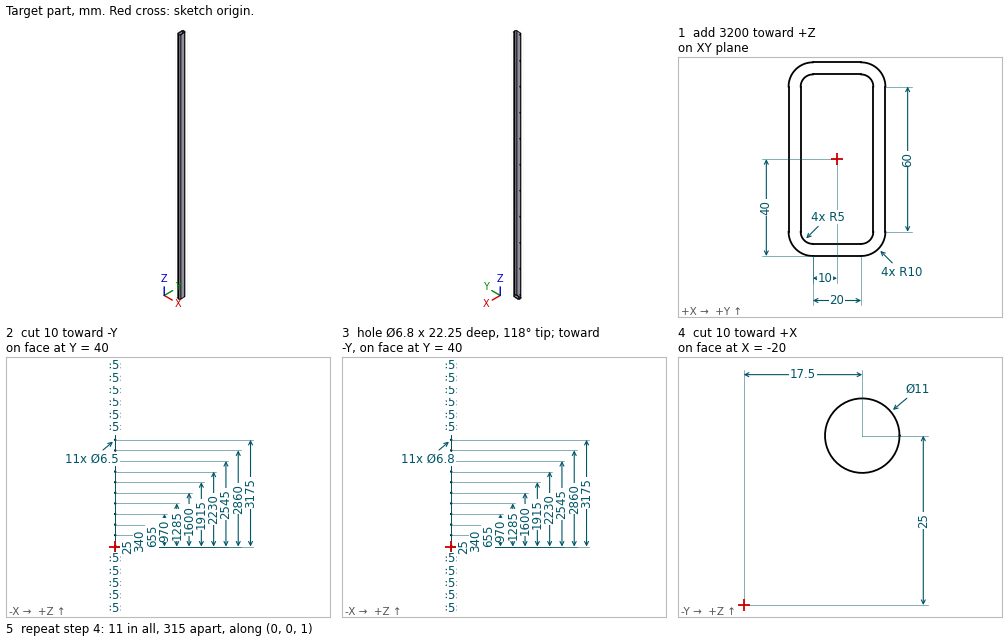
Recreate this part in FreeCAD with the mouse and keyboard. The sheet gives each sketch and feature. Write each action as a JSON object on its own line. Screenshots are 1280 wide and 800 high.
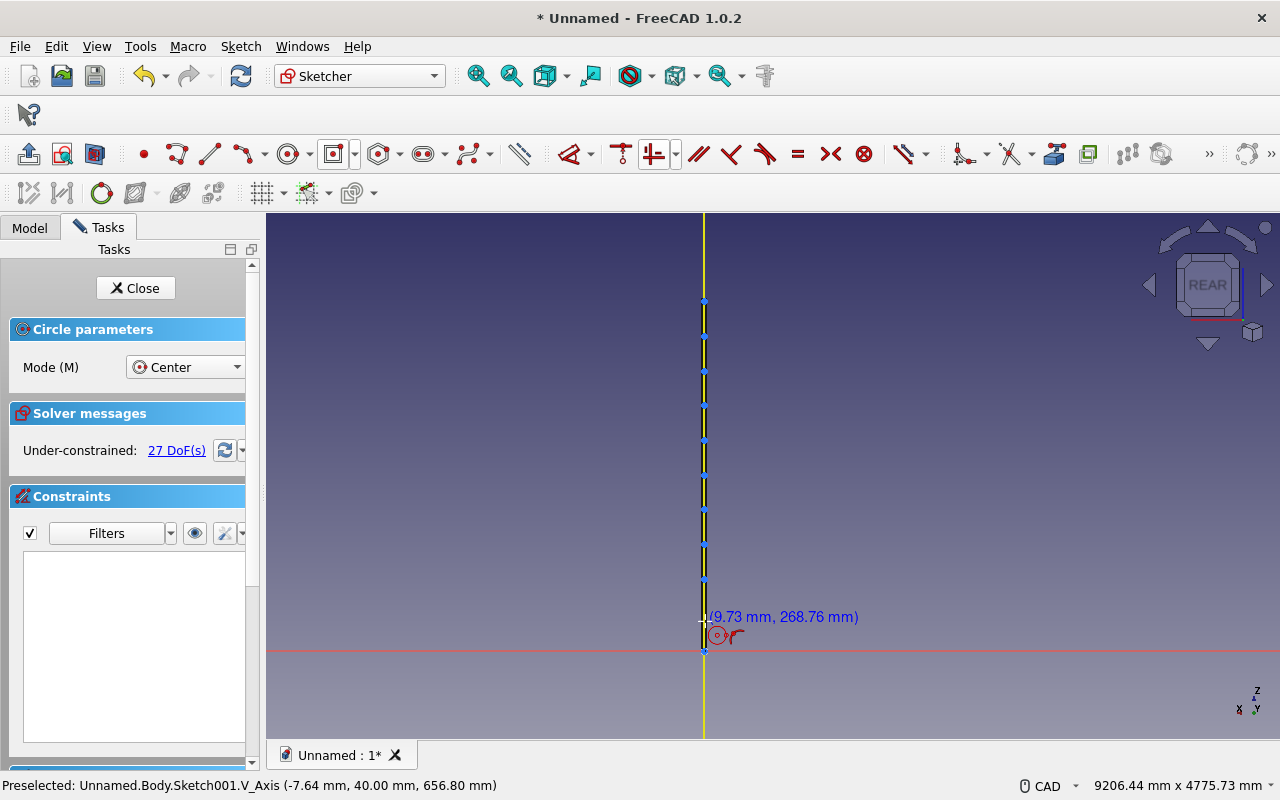
{"action": "scroll", "coordinate": [705, 614], "scroll_direction": "up", "scroll_amount": 21}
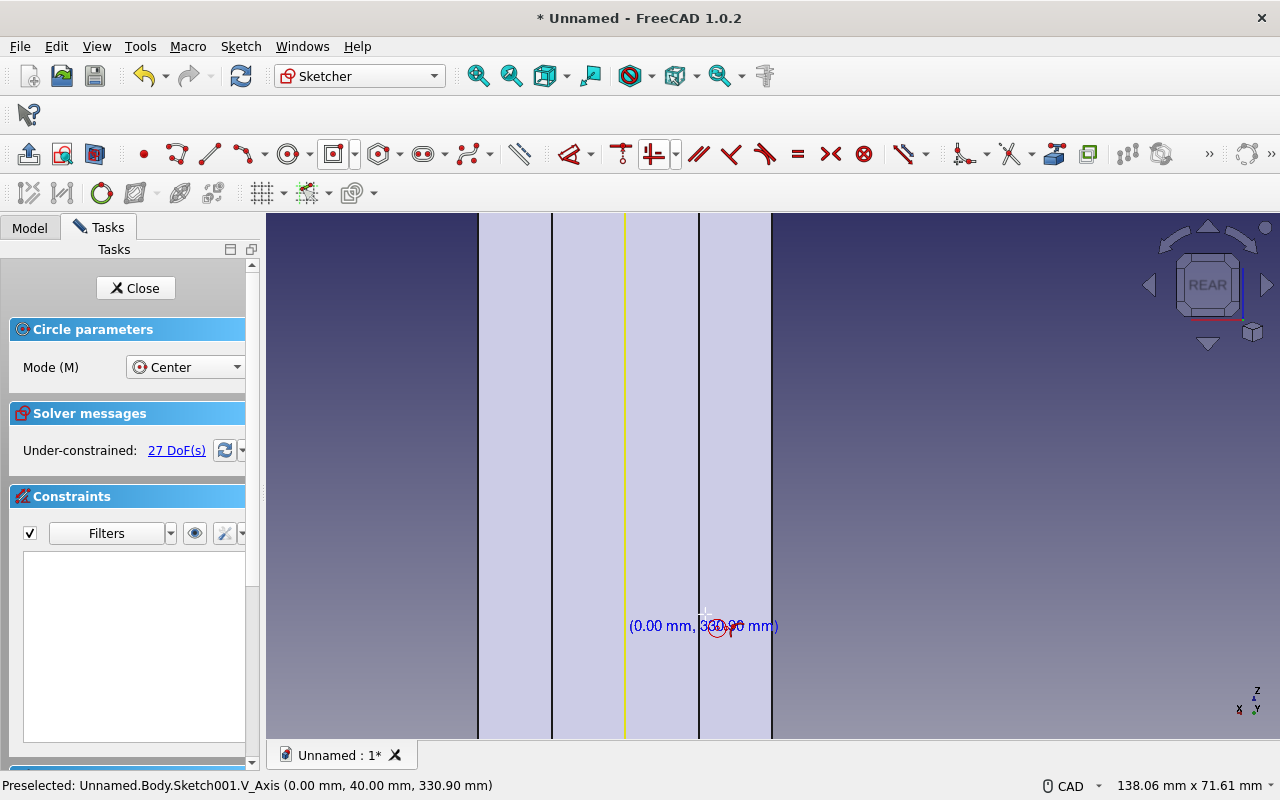
{"action": "left_click", "coordinate": [662, 564]}
{"action": "left_click", "coordinate": [679, 547]}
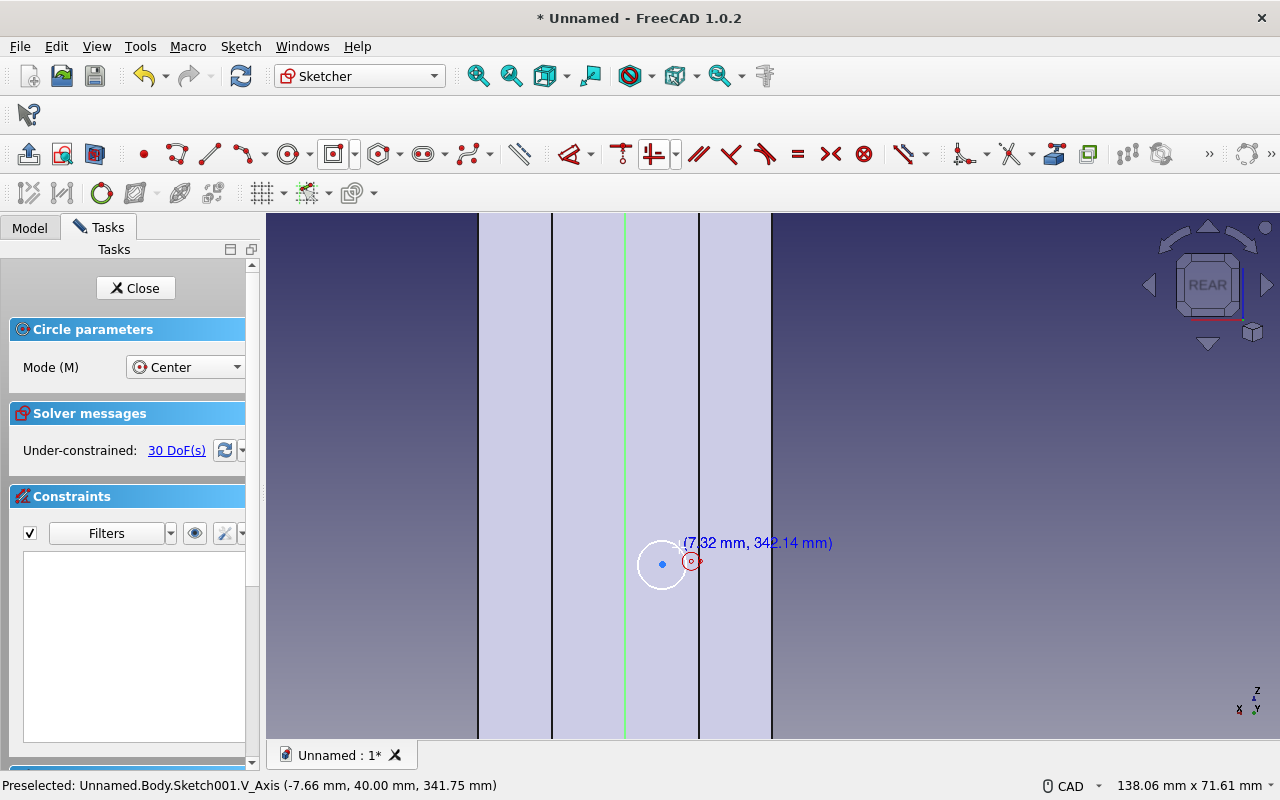
{"action": "scroll", "coordinate": [704, 476], "scroll_direction": "down", "scroll_amount": 15}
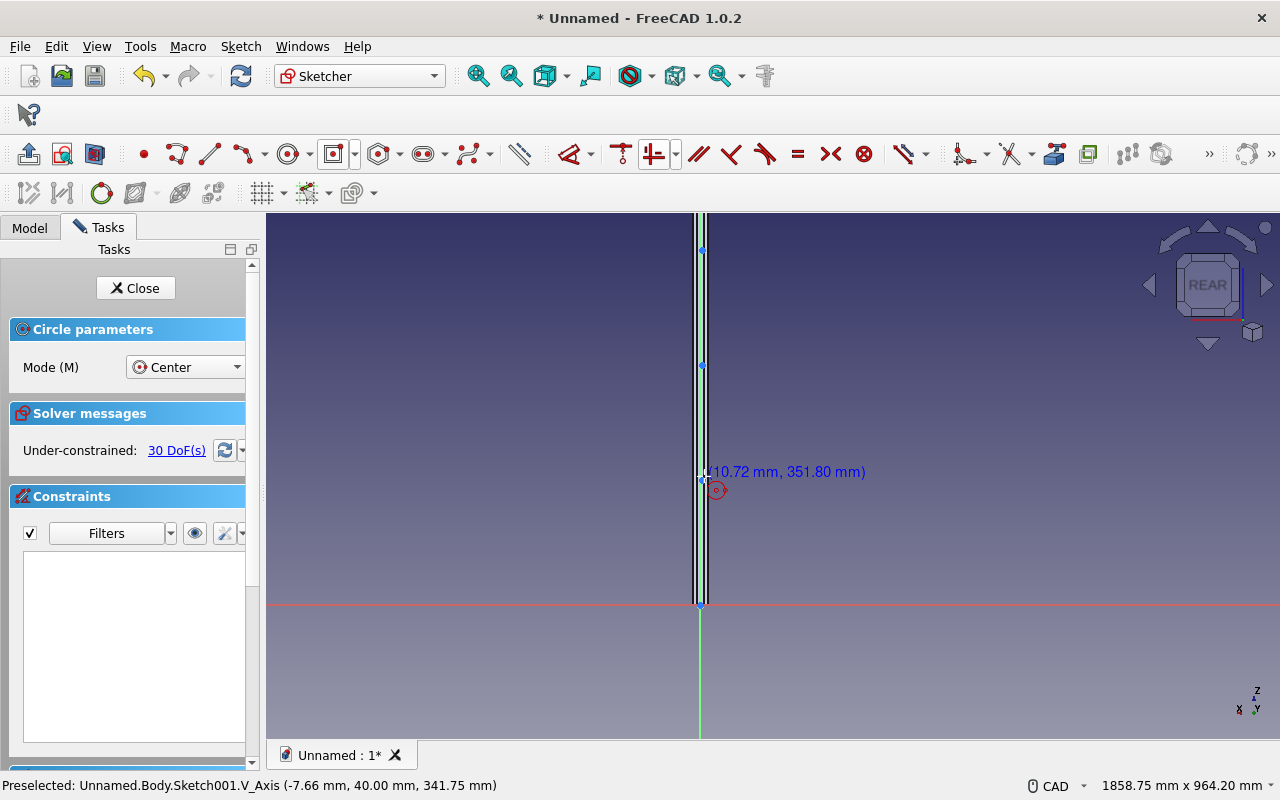
{"action": "scroll", "coordinate": [706, 671], "scroll_direction": "down", "scroll_amount": 6}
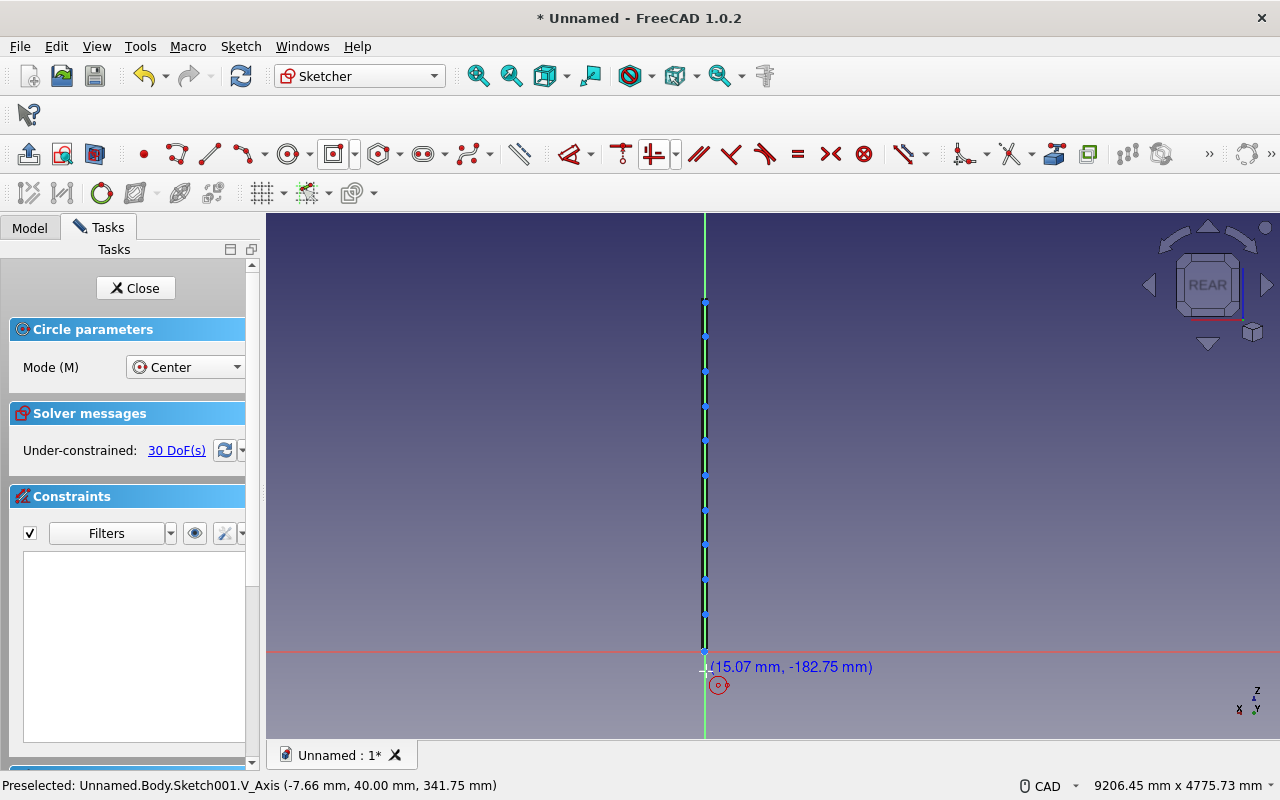
{"action": "scroll", "coordinate": [705, 649], "scroll_direction": "up", "scroll_amount": 21}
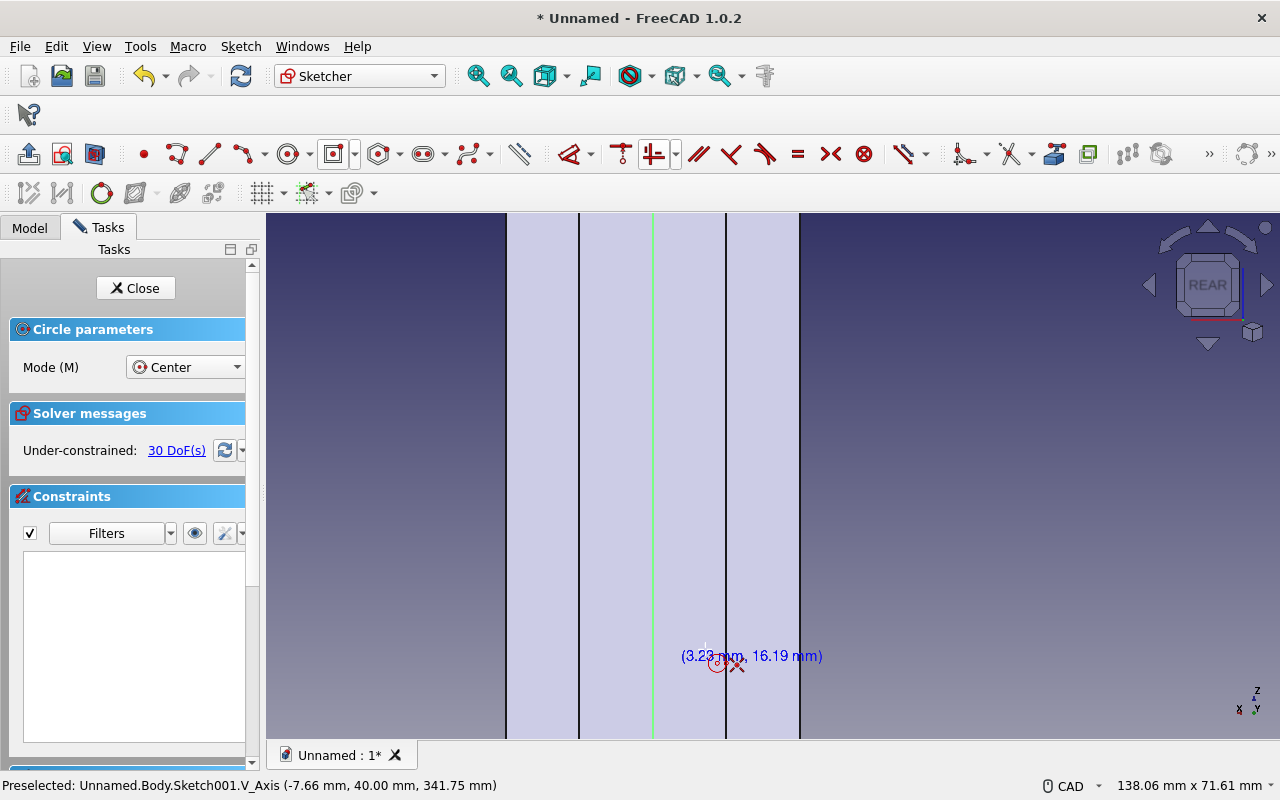
{"action": "left_click", "coordinate": [690, 596]}
{"action": "left_click", "coordinate": [706, 580]}
{"action": "key", "text": "Escape"}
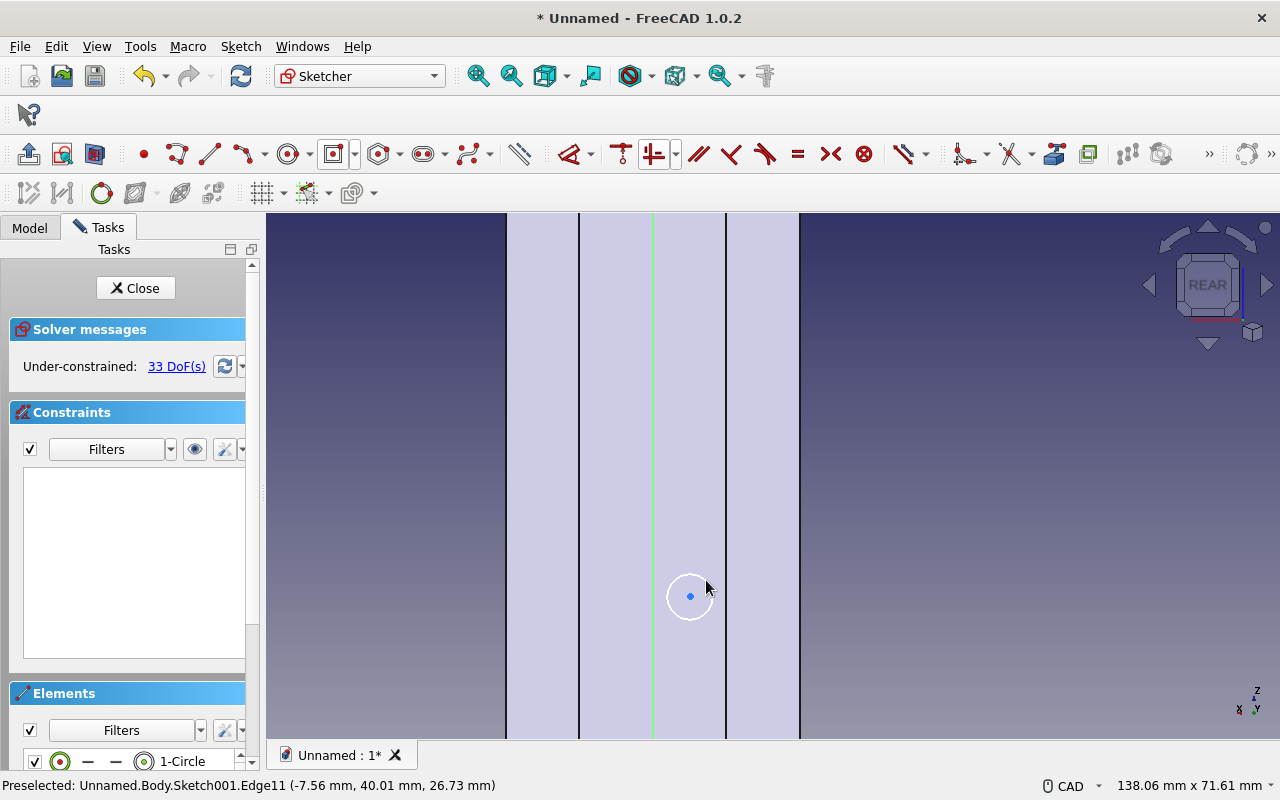
{"action": "scroll", "coordinate": [704, 476], "scroll_direction": "down", "scroll_amount": 15}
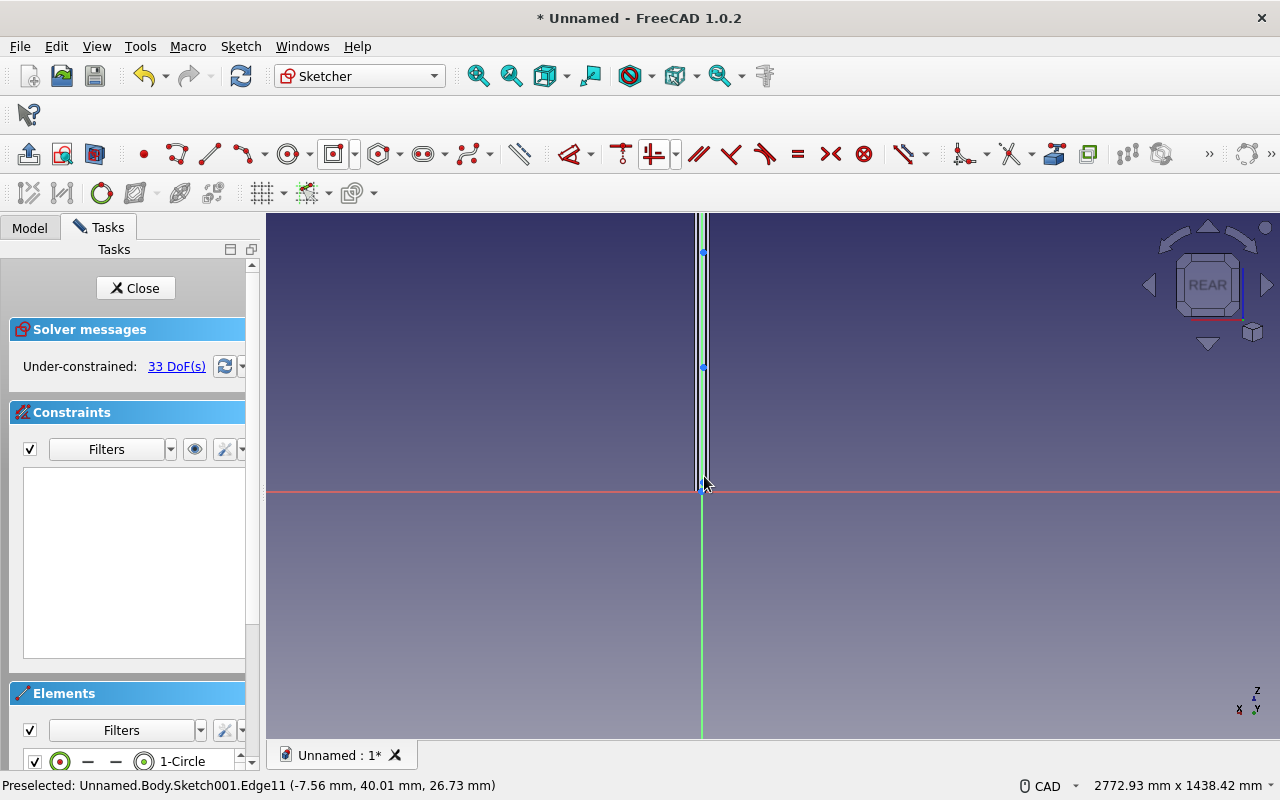
{"action": "scroll", "coordinate": [705, 711], "scroll_direction": "down", "scroll_amount": 6}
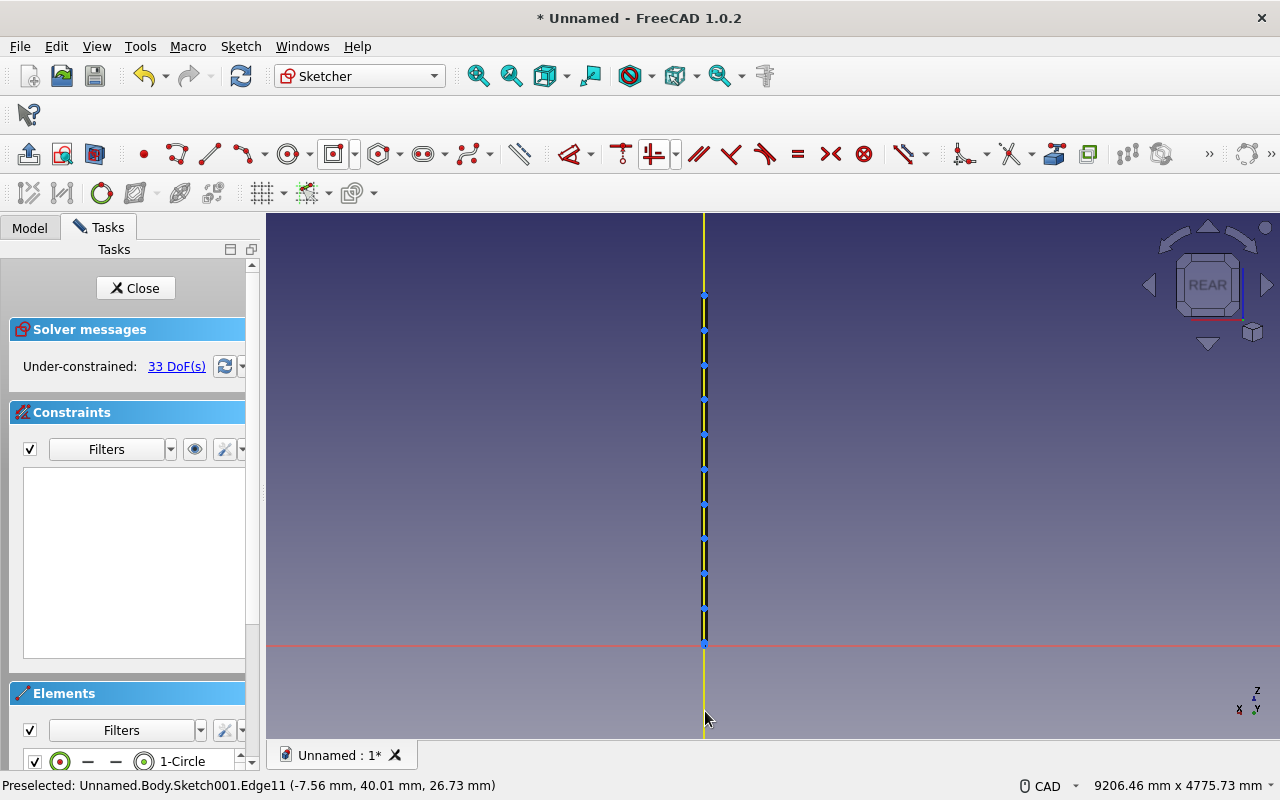
{"action": "scroll", "coordinate": [705, 296], "scroll_direction": "up", "scroll_amount": 14}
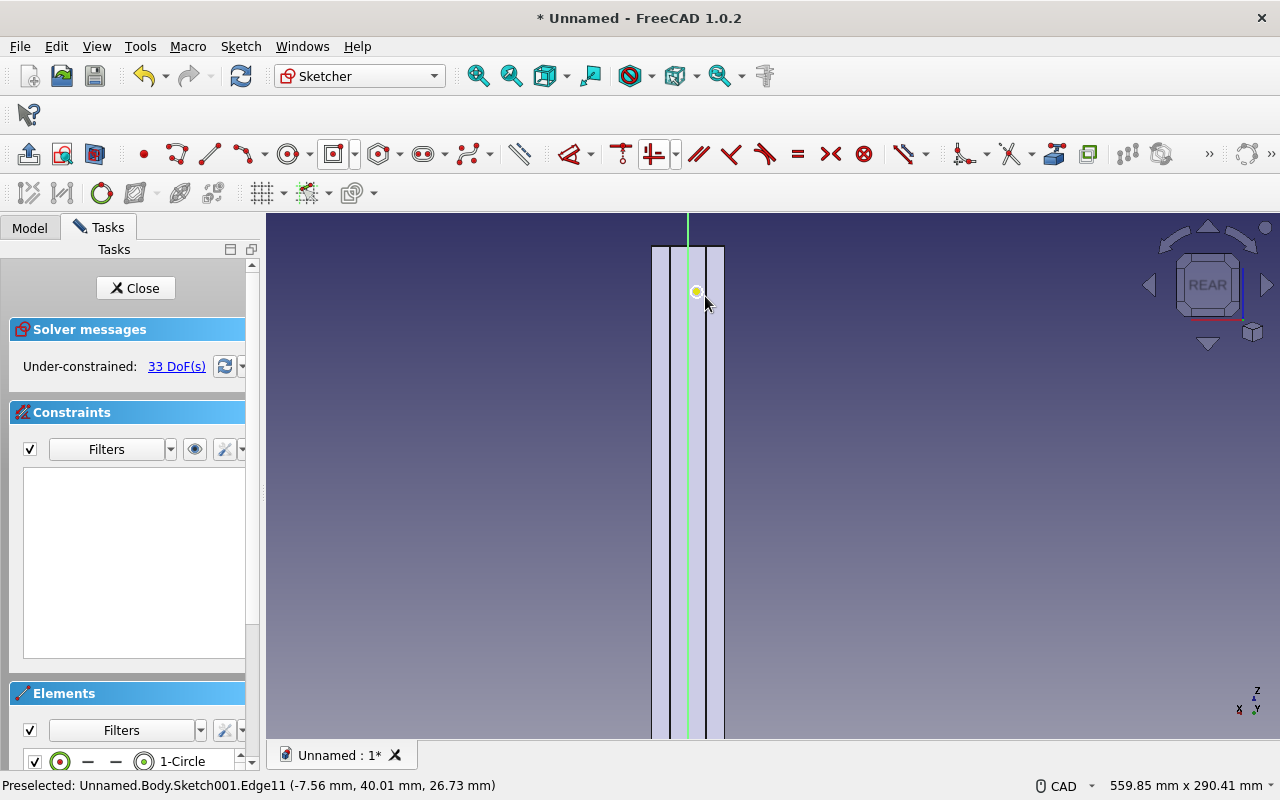
{"action": "left_click", "coordinate": [701, 288]}